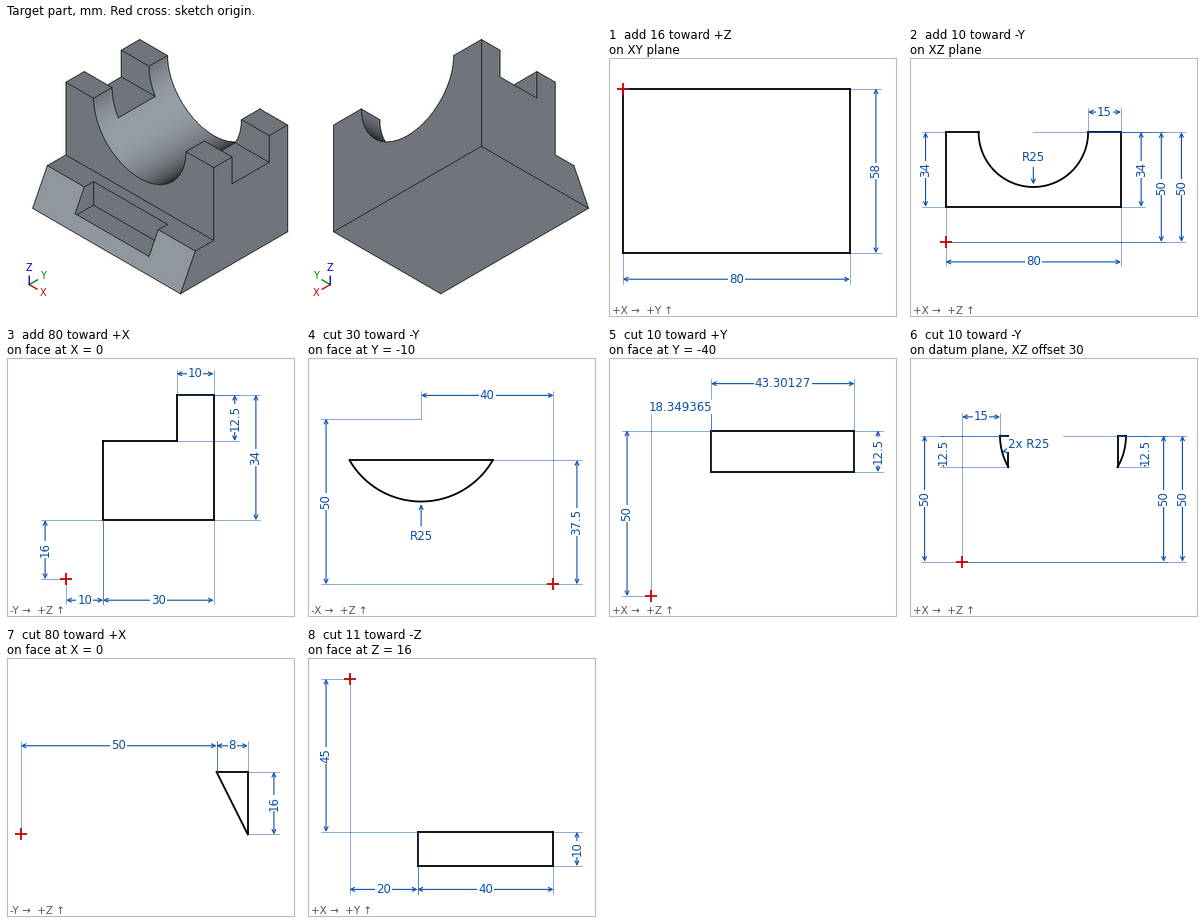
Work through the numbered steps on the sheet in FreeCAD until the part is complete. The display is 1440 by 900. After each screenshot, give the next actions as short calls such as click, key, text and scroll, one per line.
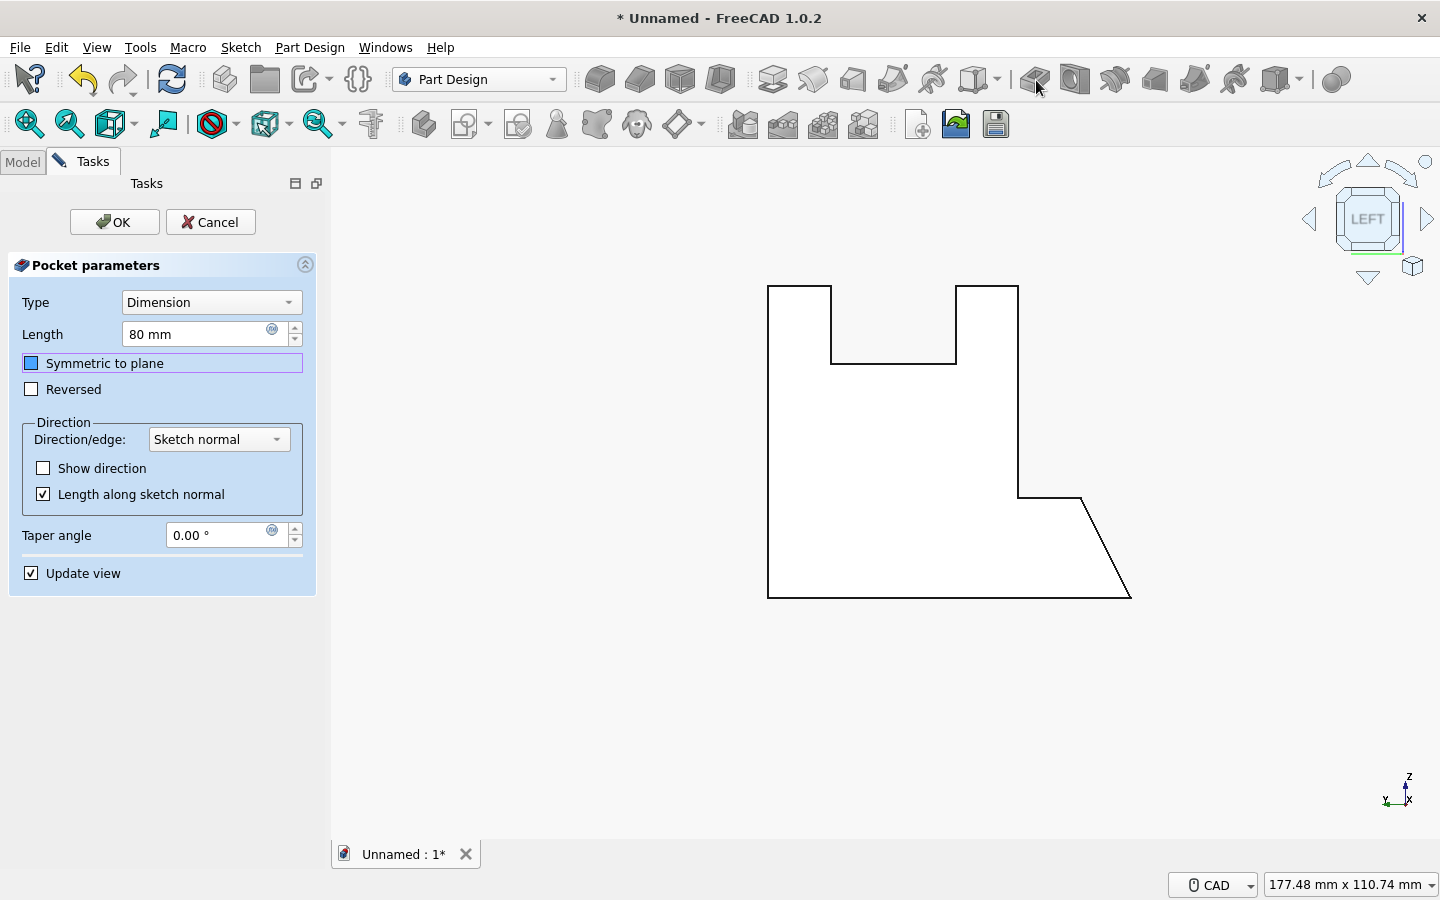
click(115, 222)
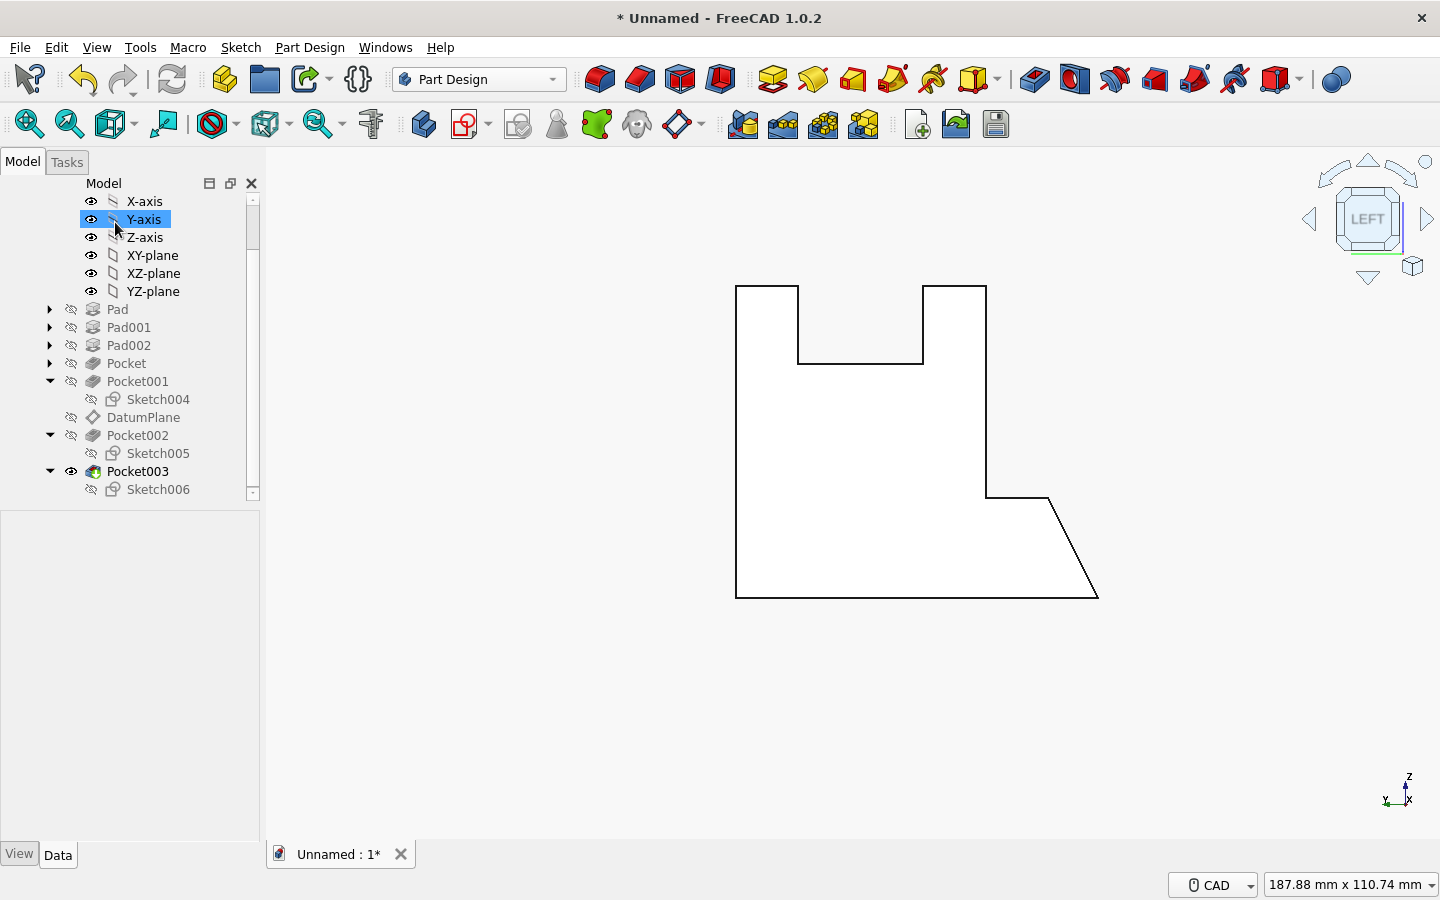
key(0)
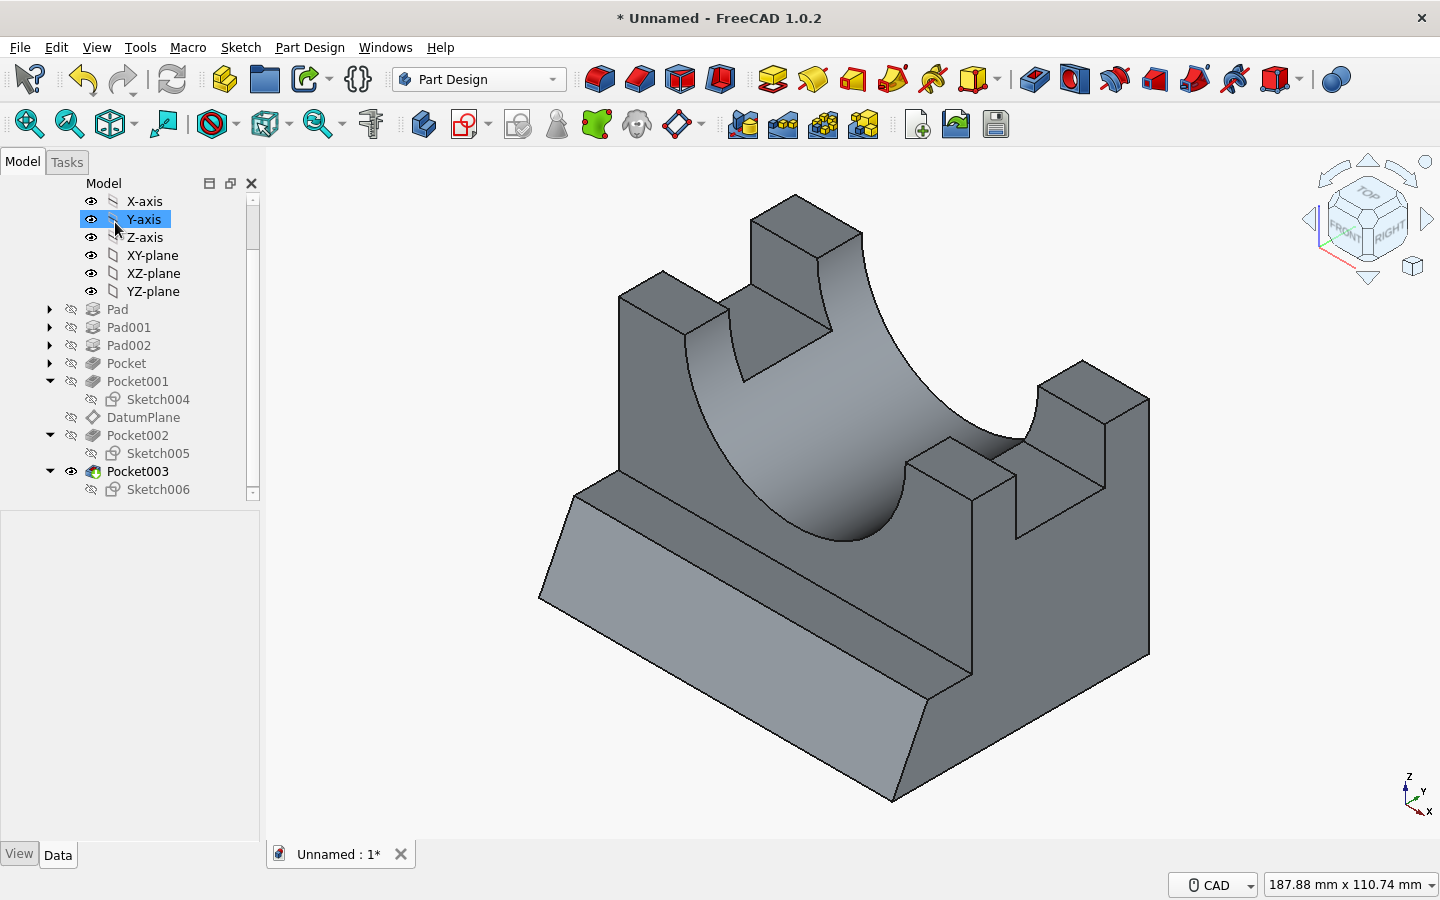
click(925, 671)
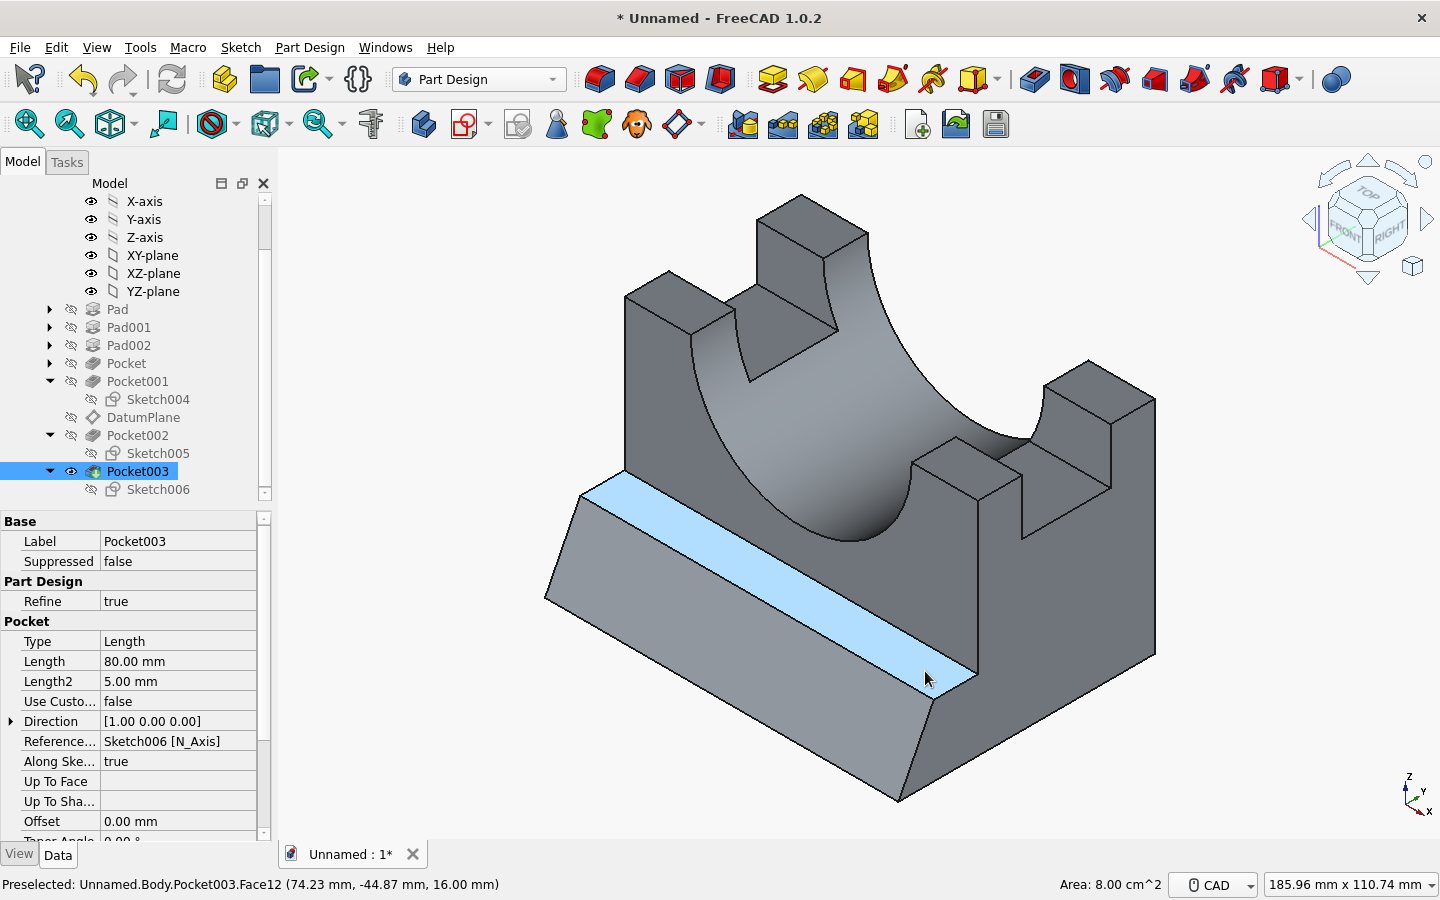
click(464, 124)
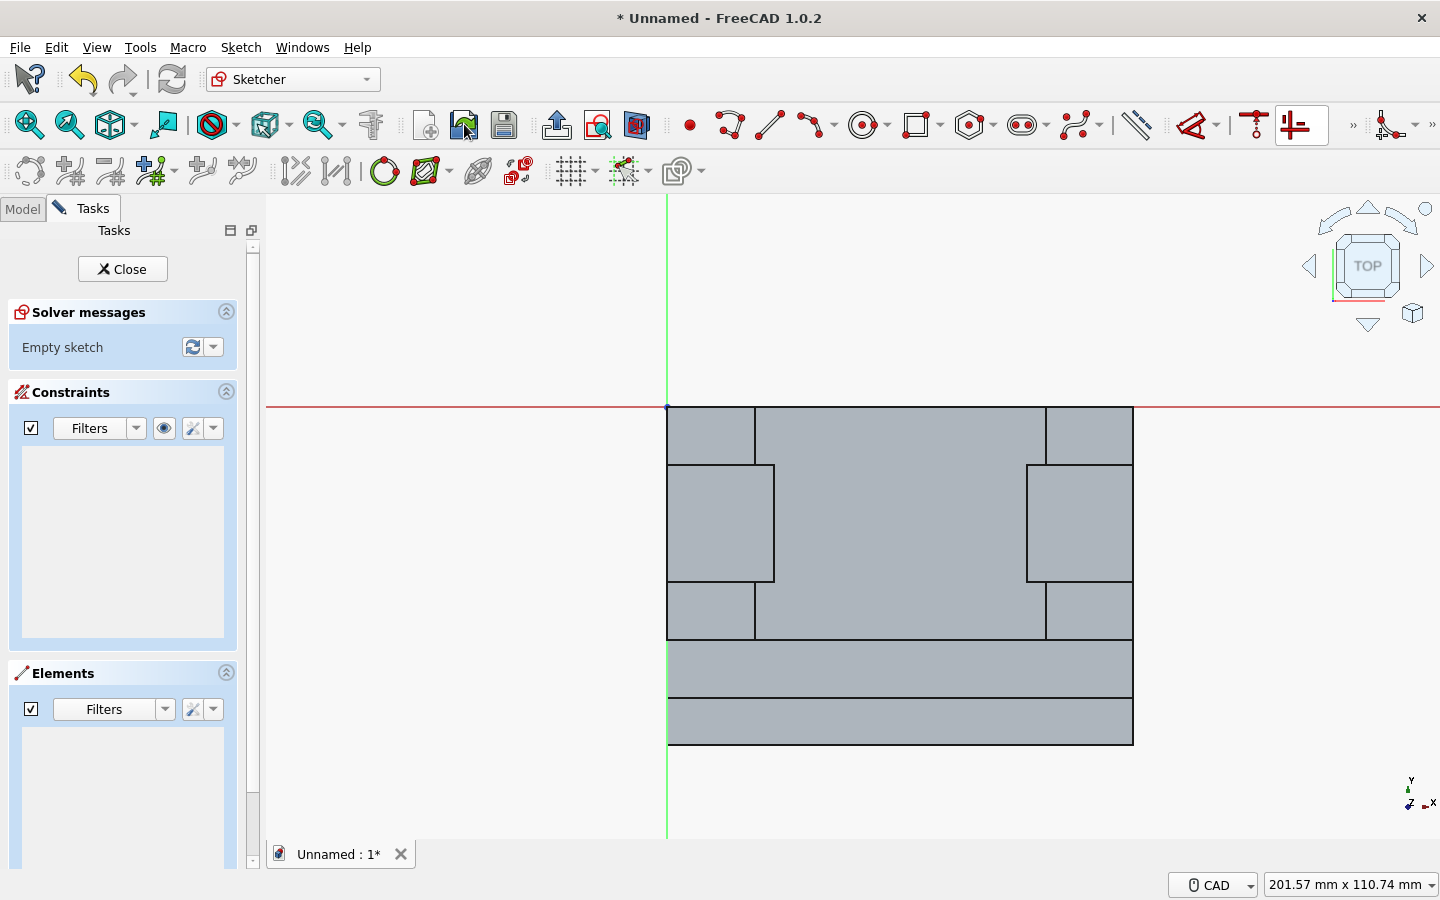
click(638, 126)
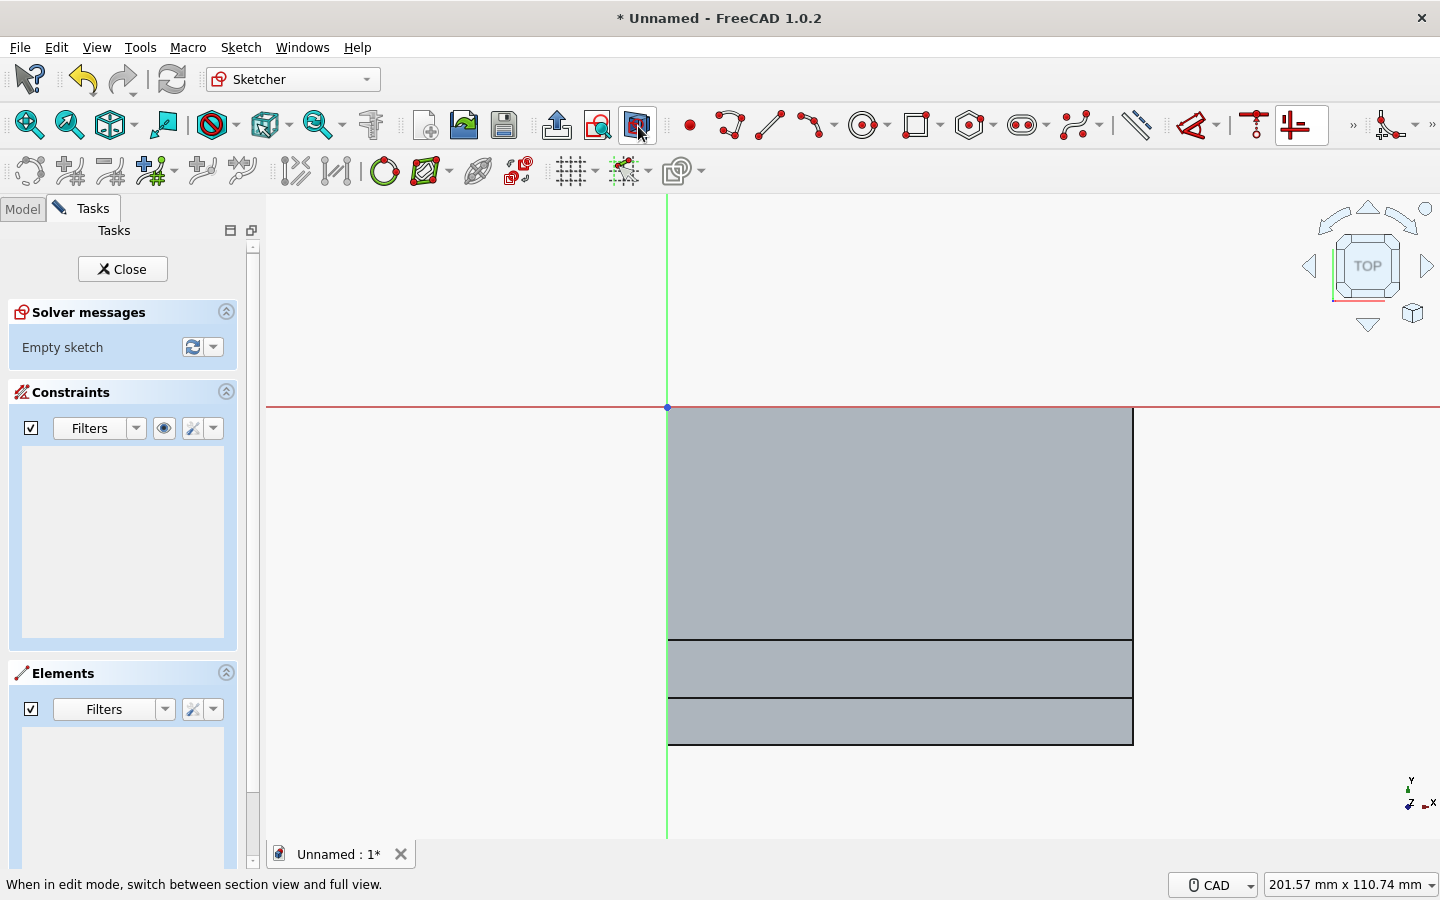
click(916, 126)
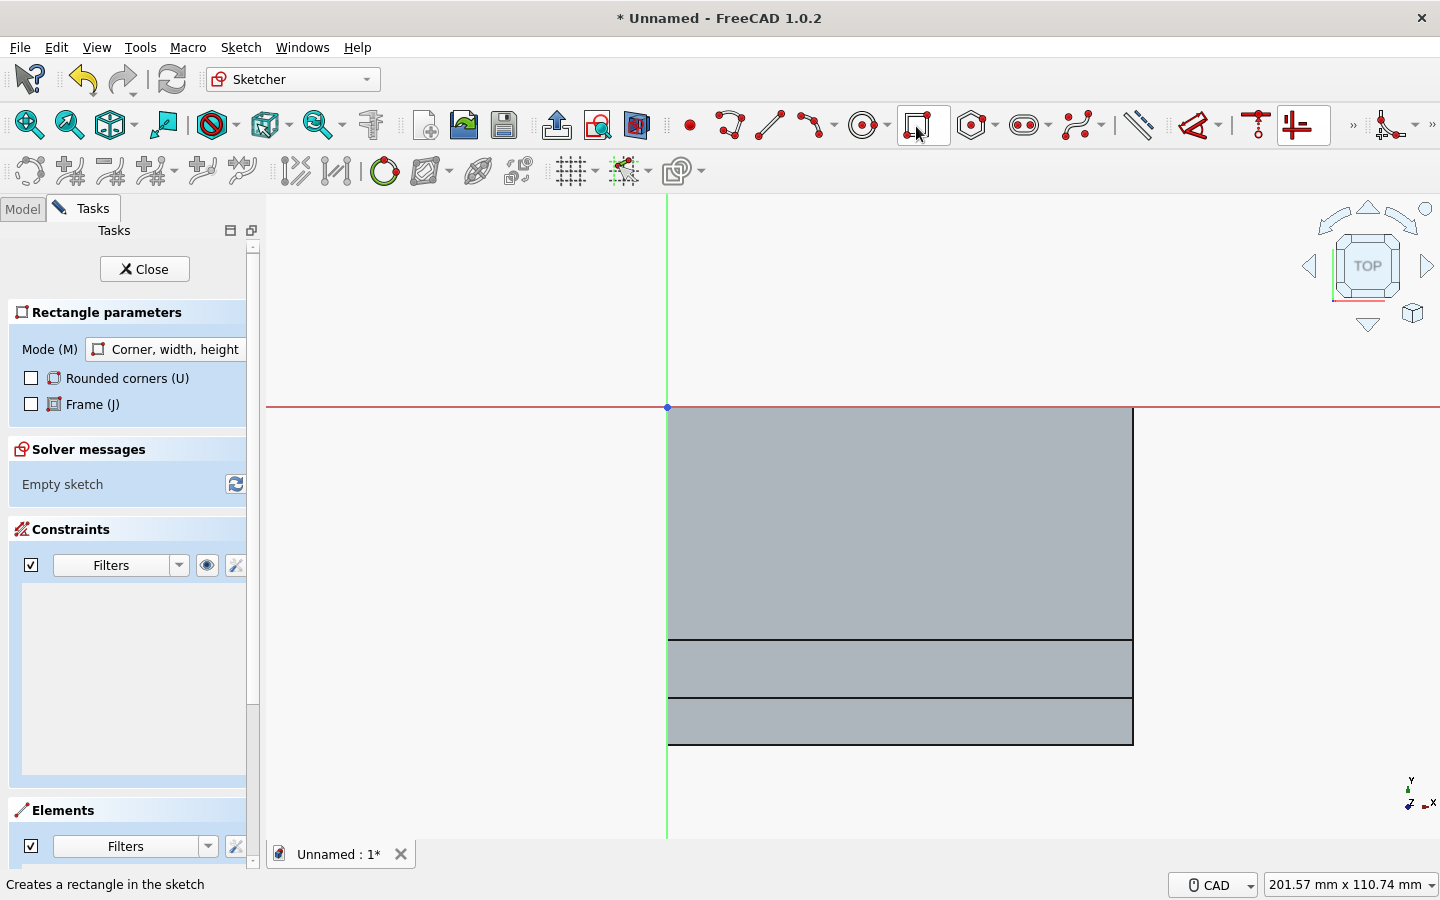
click(784, 669)
move(1017, 727)